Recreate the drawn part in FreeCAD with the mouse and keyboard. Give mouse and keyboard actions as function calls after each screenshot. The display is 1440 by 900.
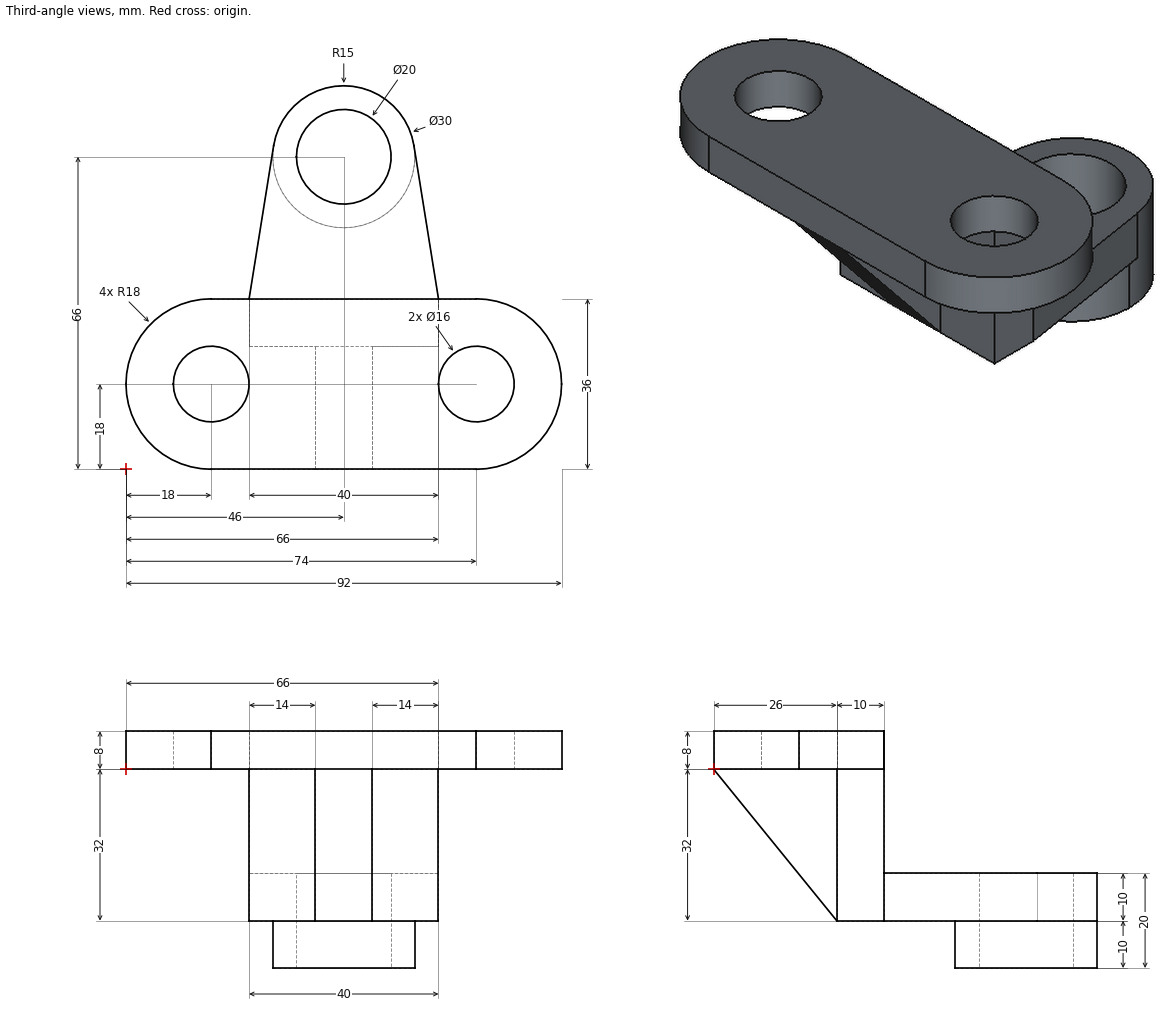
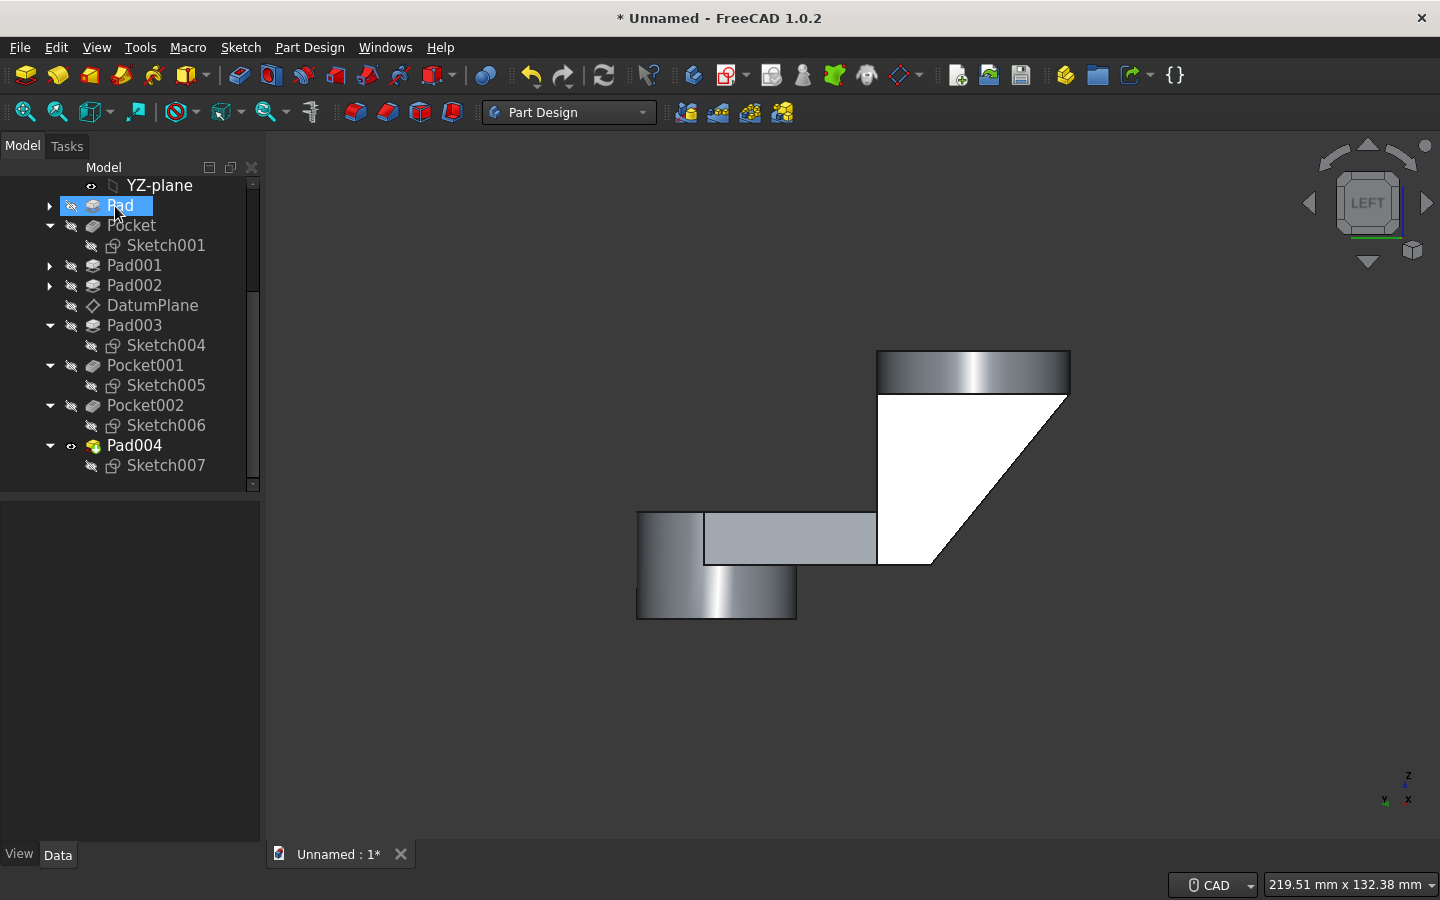
click(26, 112)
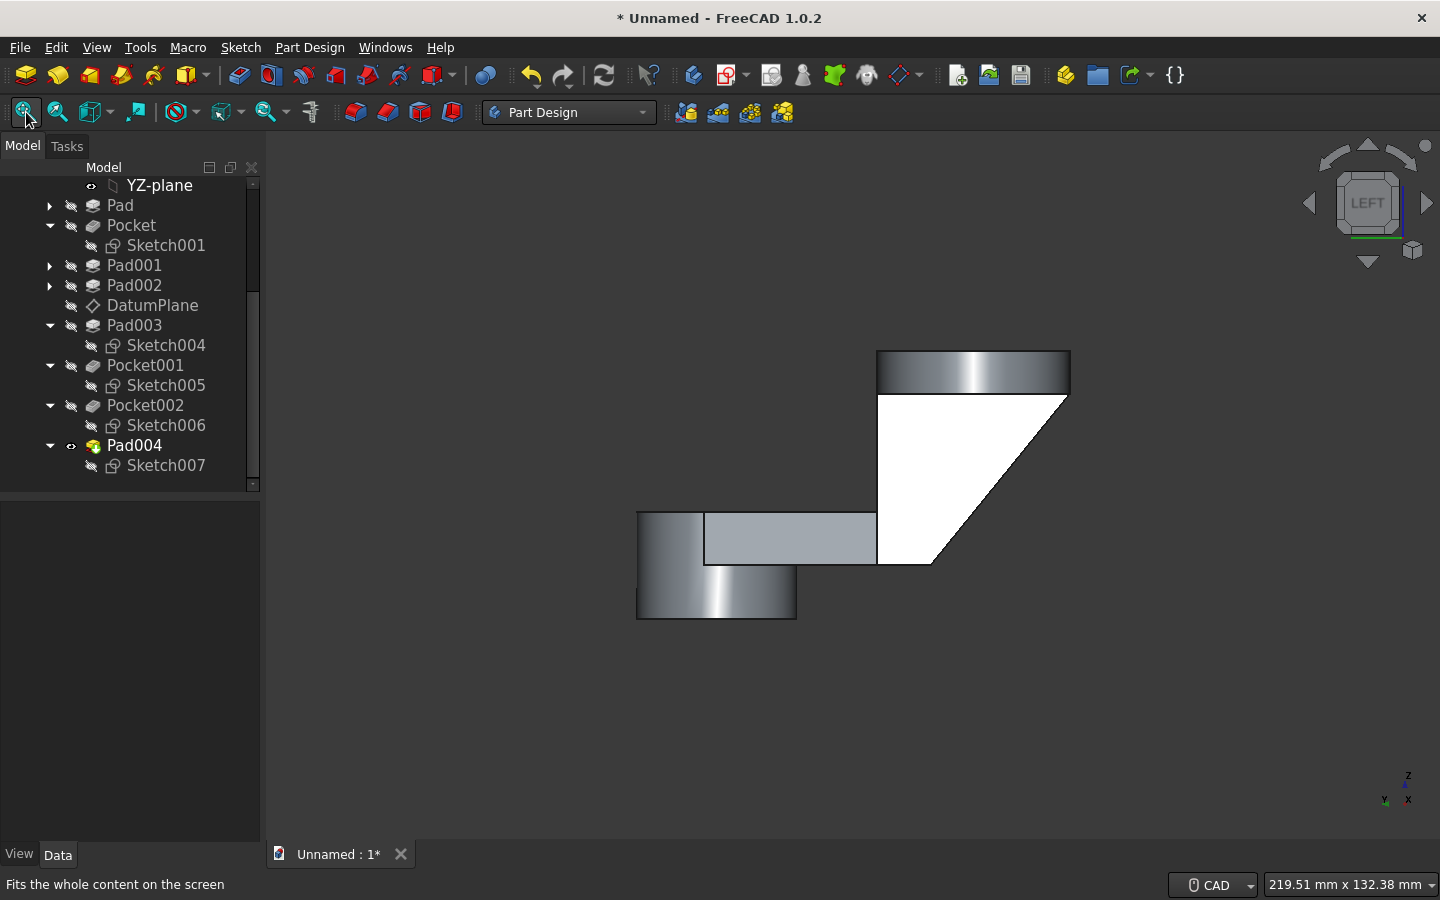
click(946, 454)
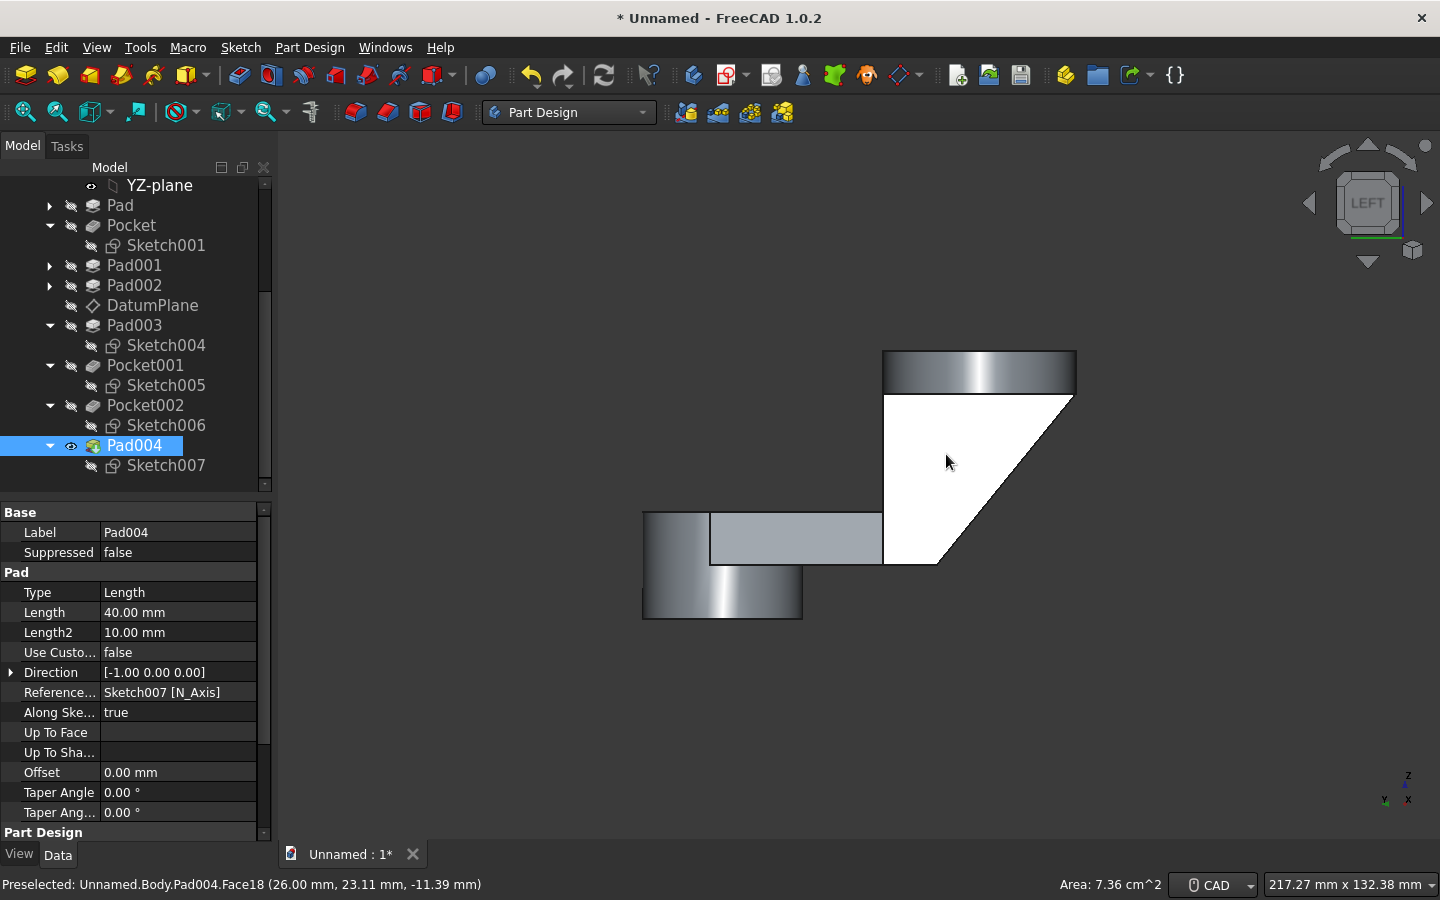
click(726, 76)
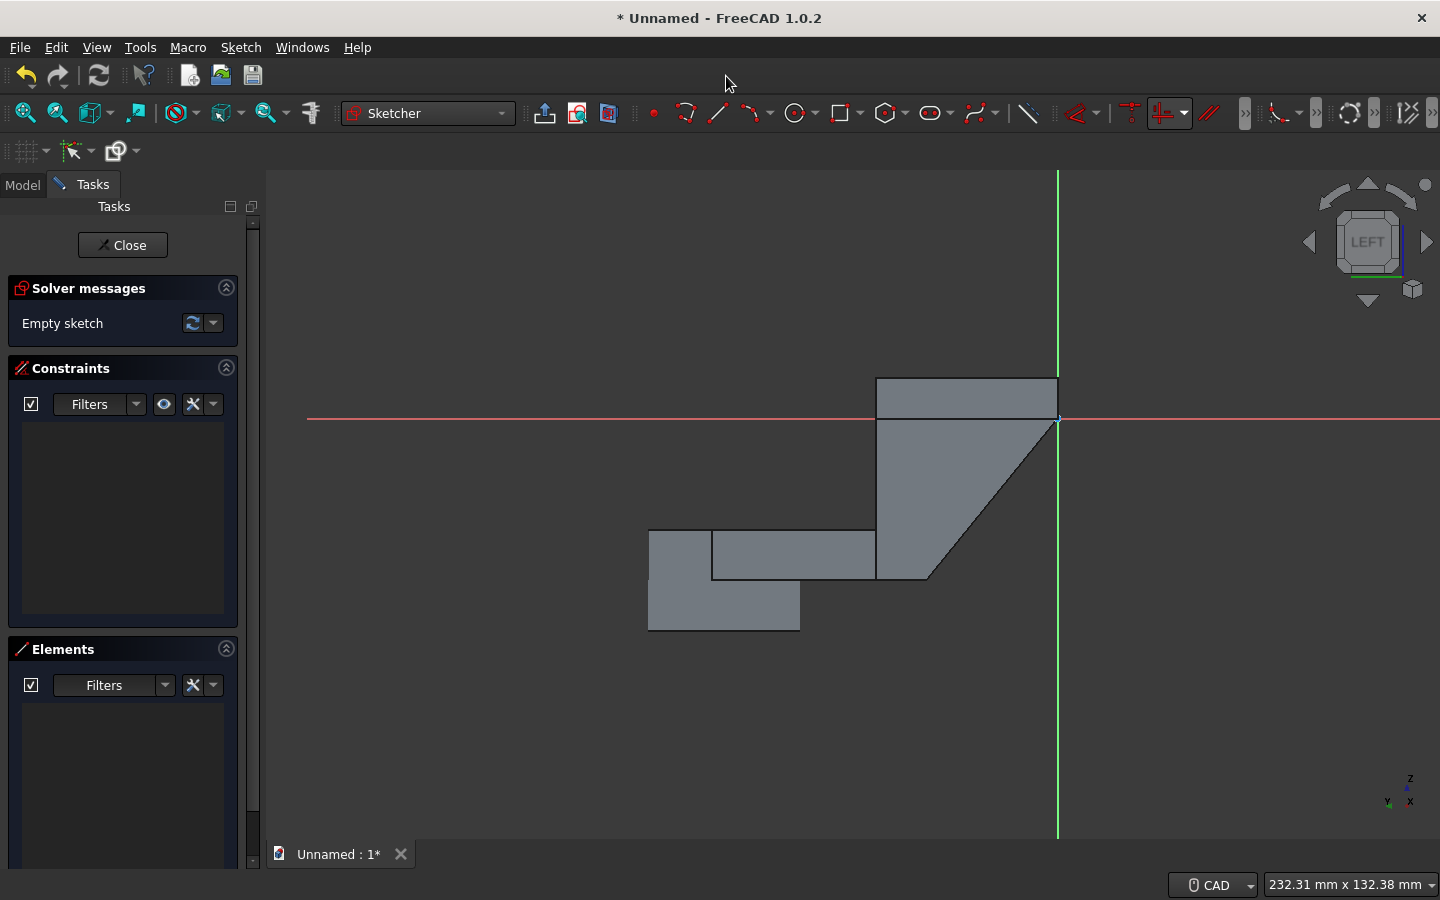
scroll(1113, 497, up, 5)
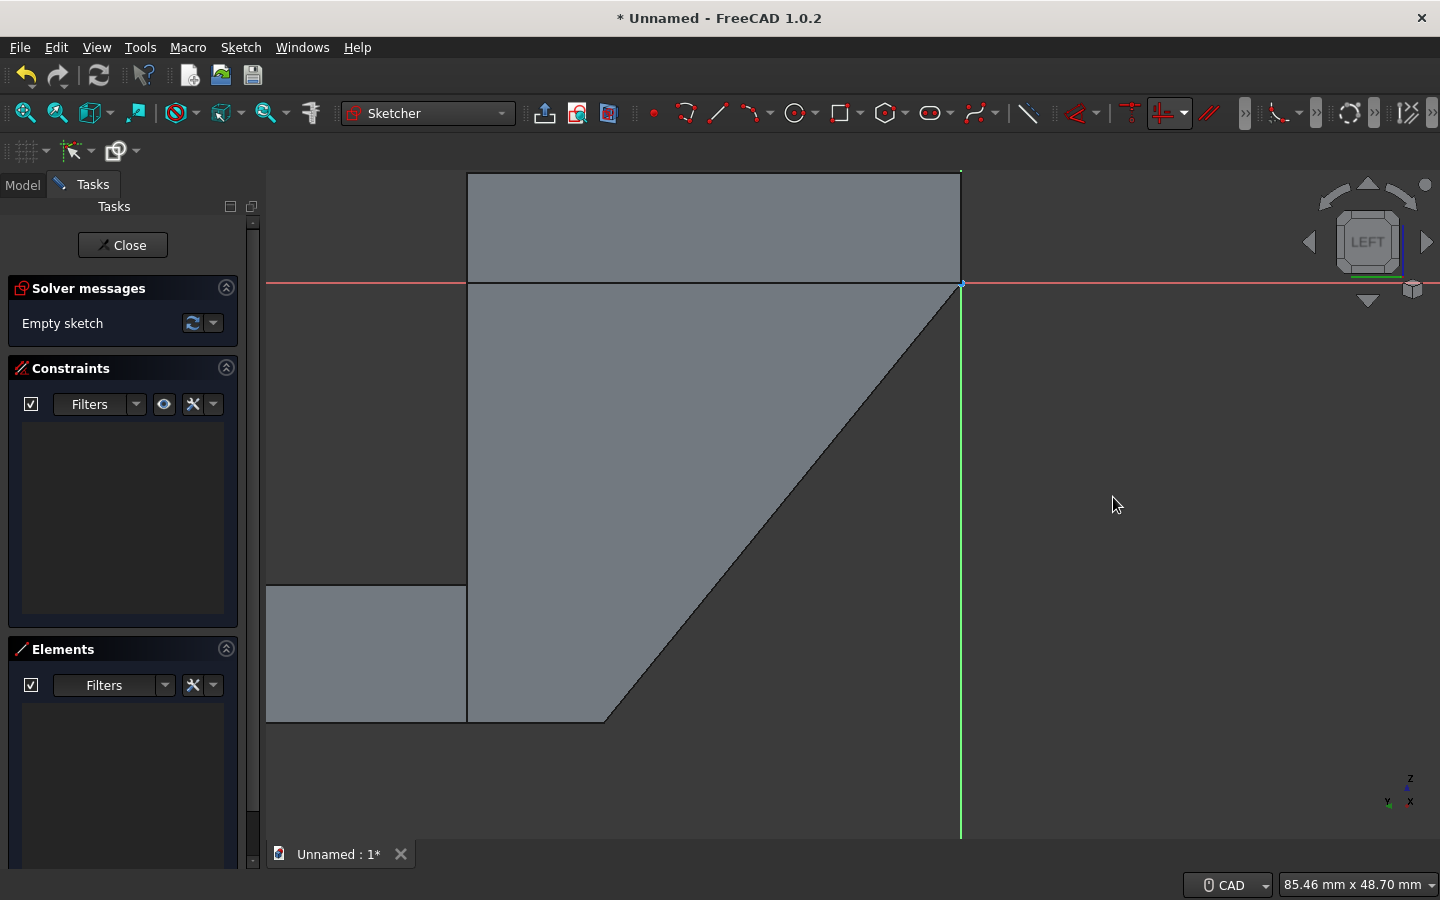
click(686, 114)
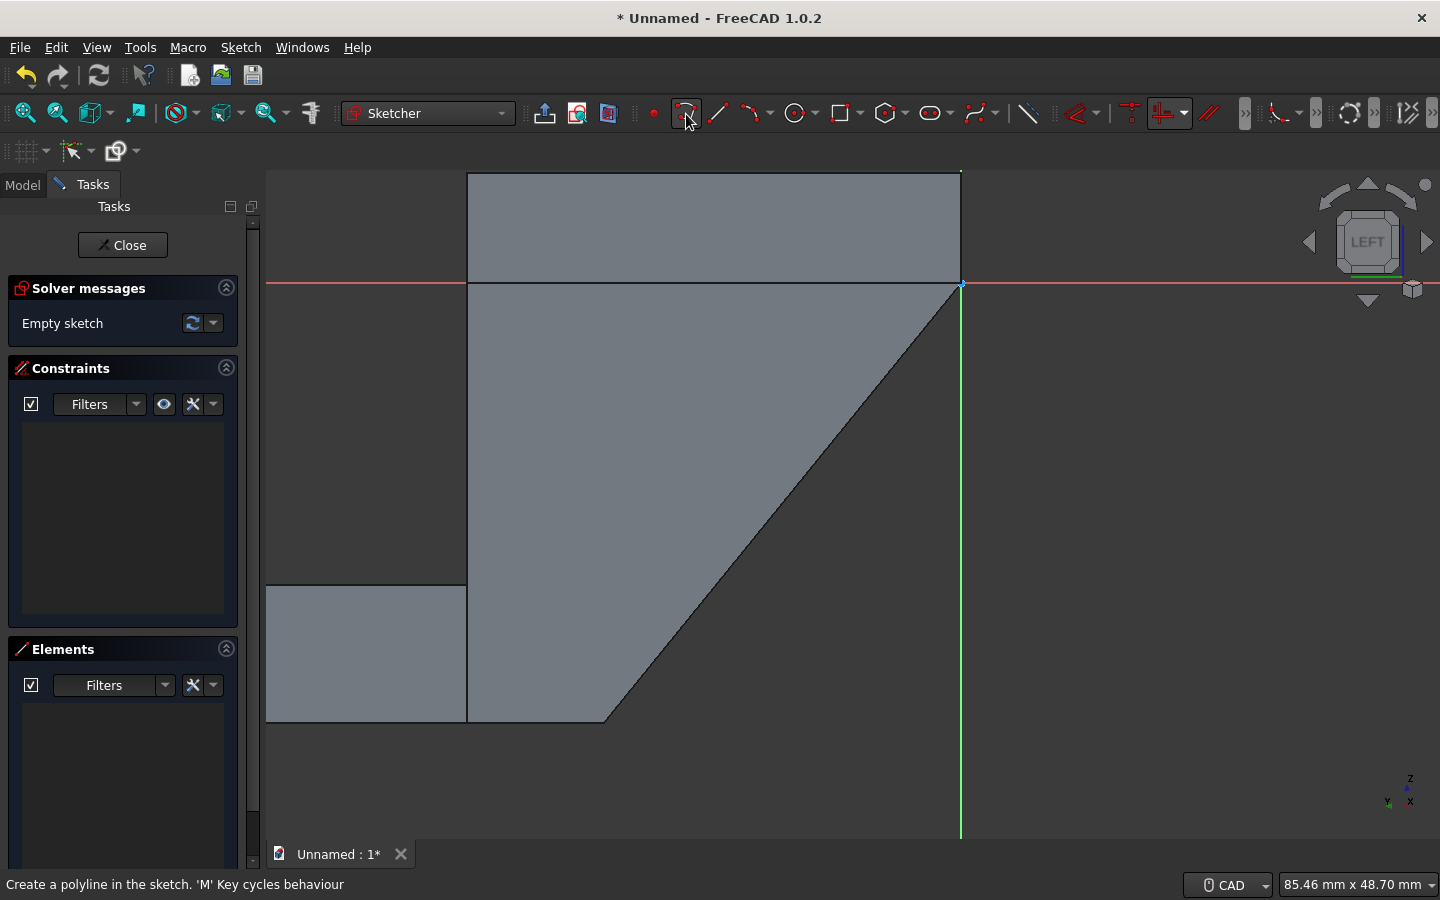
click(961, 283)
click(604, 292)
click(604, 723)
click(961, 283)
key(Escape)
key(Escape)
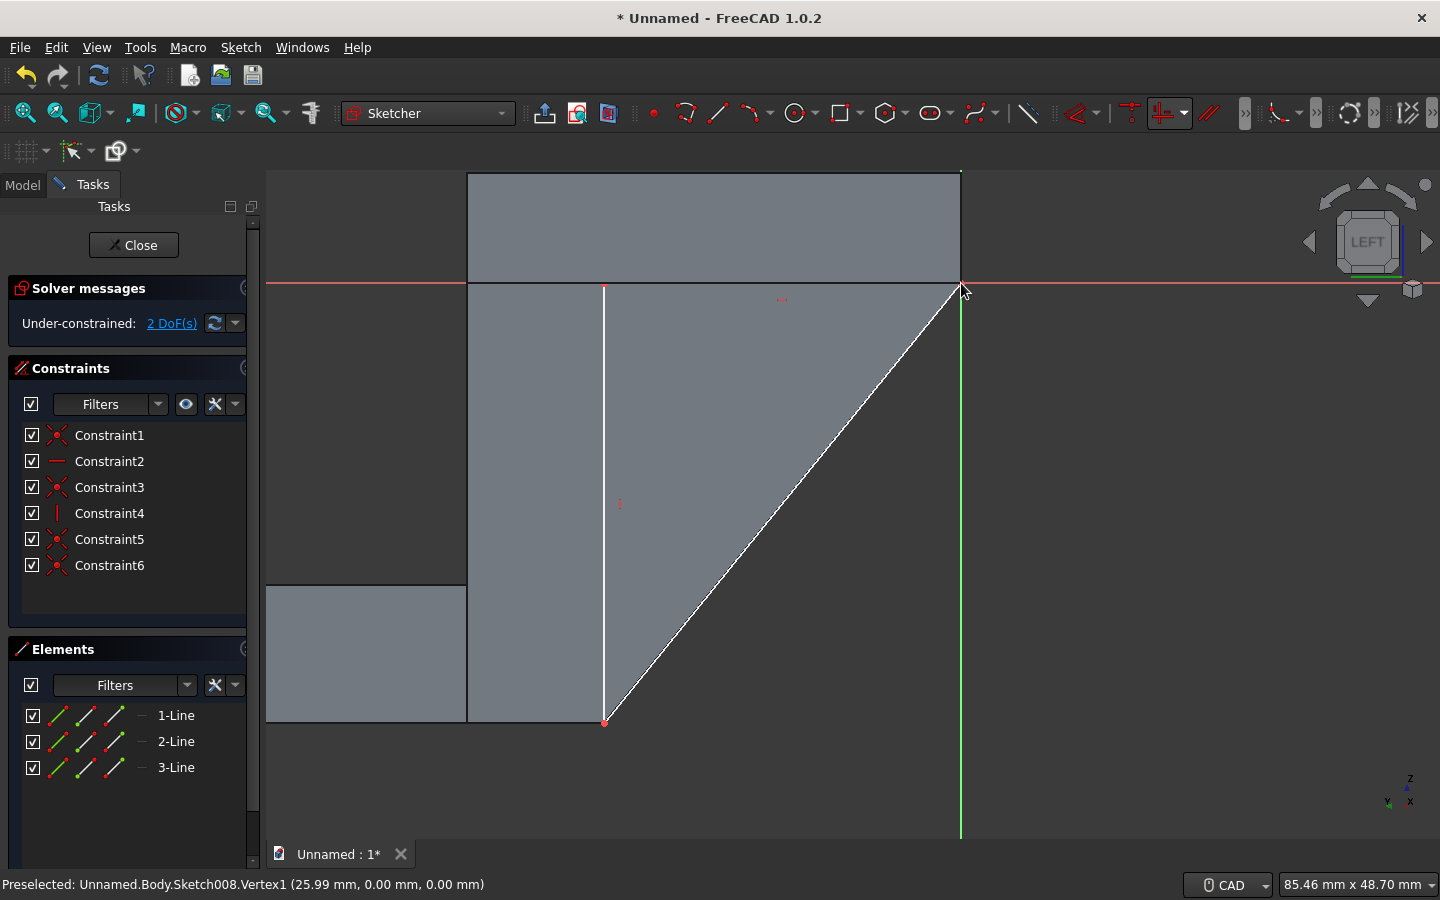
click(1076, 114)